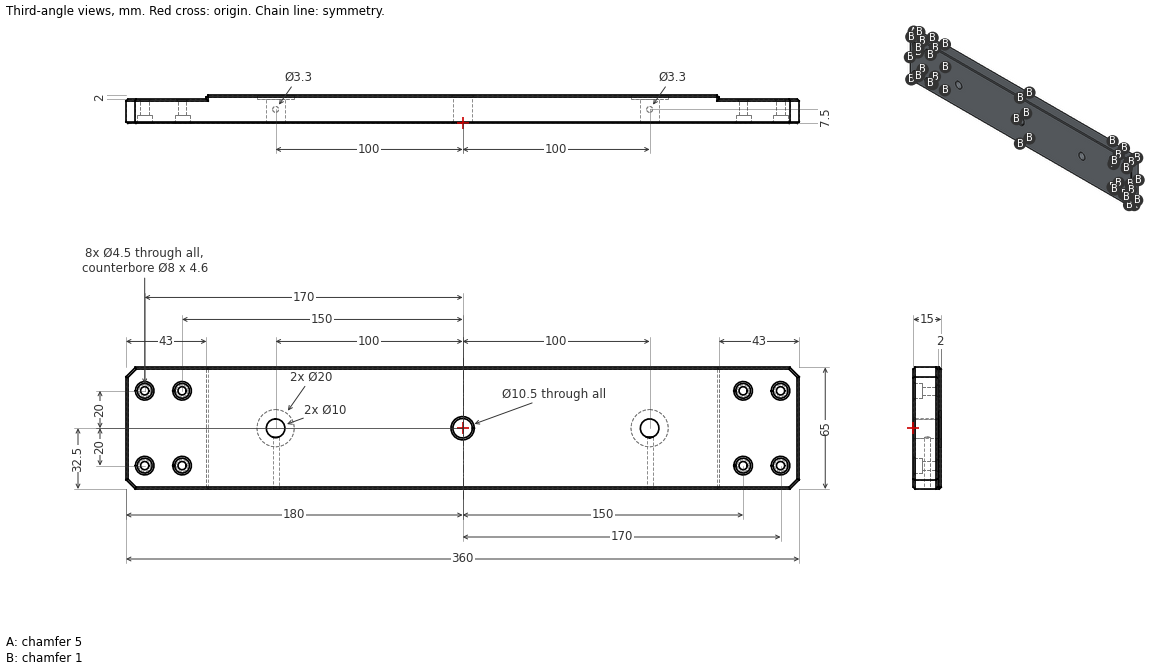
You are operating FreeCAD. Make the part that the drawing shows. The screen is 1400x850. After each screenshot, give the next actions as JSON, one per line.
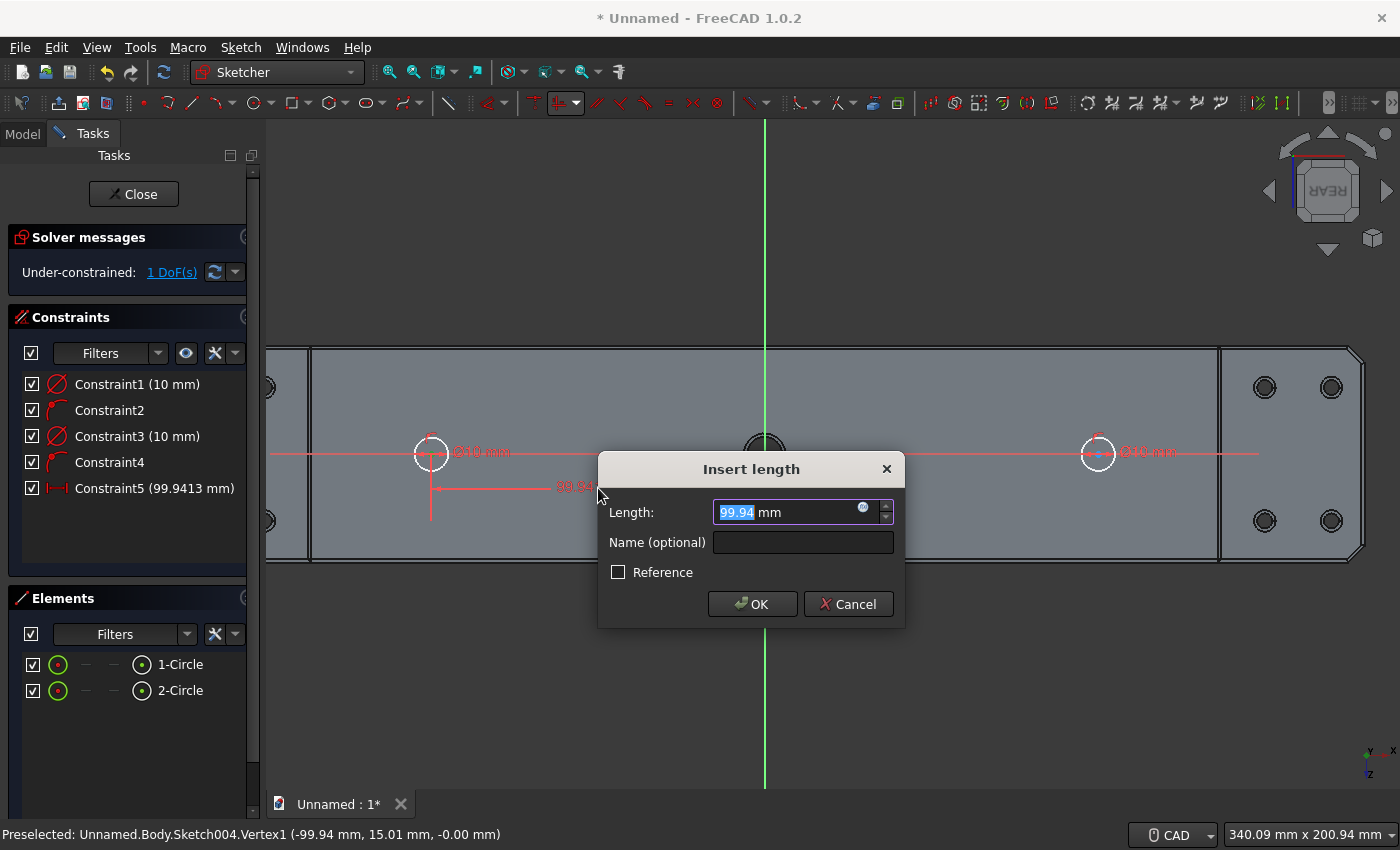
{"action": "type", "text": "100"}
{"action": "key", "text": "Return"}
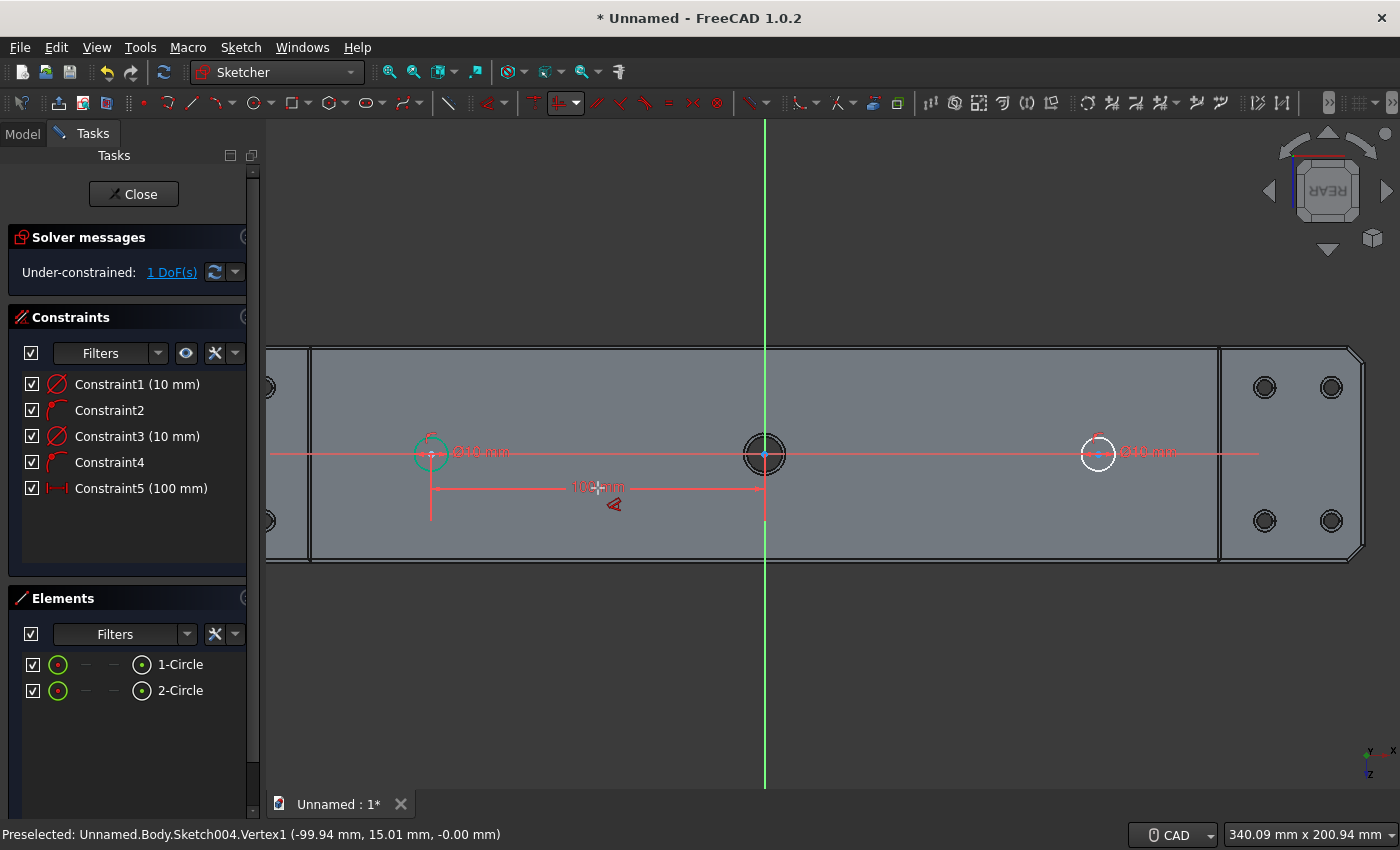
{"action": "left_click", "coordinate": [1098, 454]}
{"action": "left_click", "coordinate": [931, 488]}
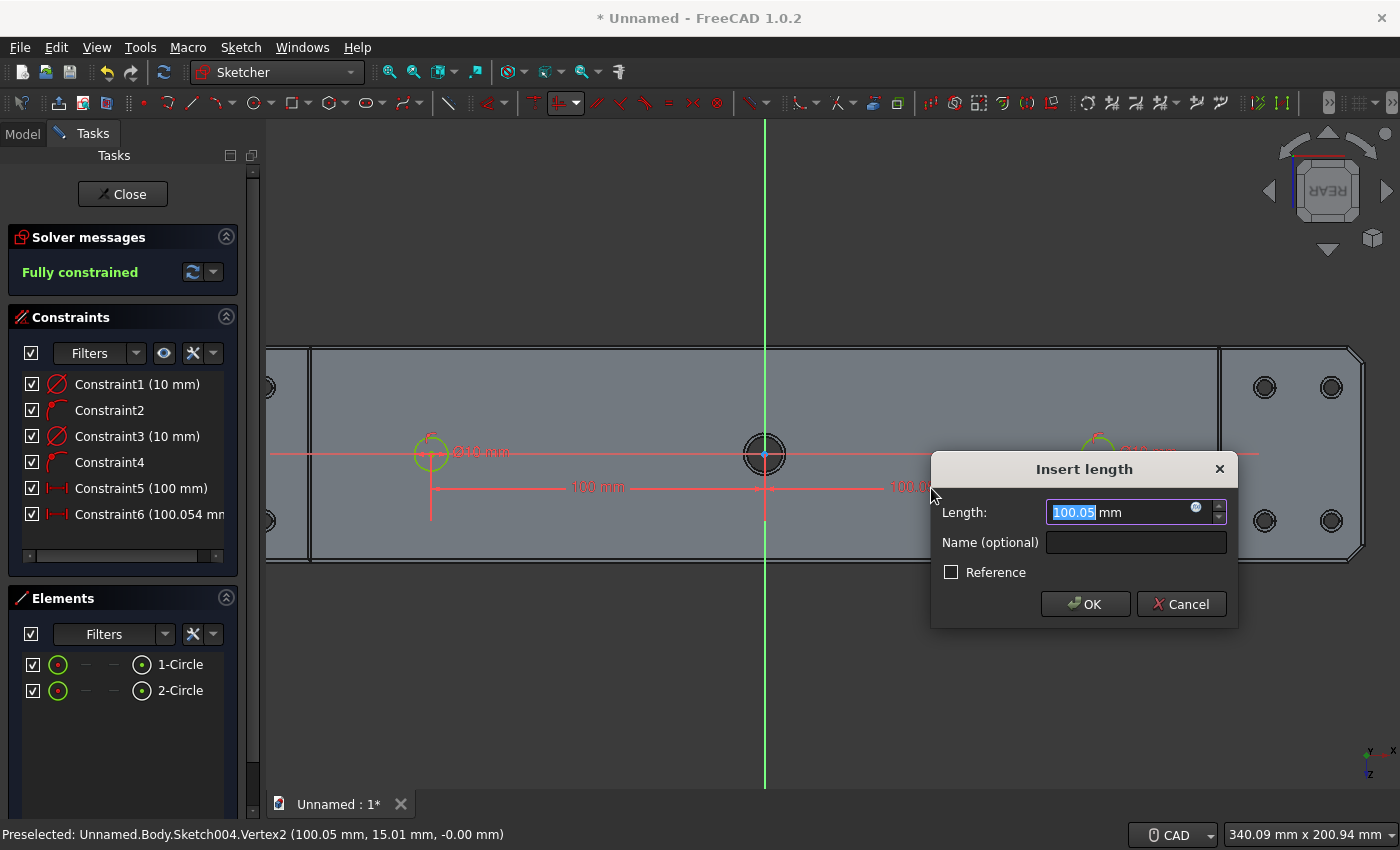
{"action": "type", "text": "100"}
{"action": "key", "text": "Return"}
{"action": "key", "text": "Escape"}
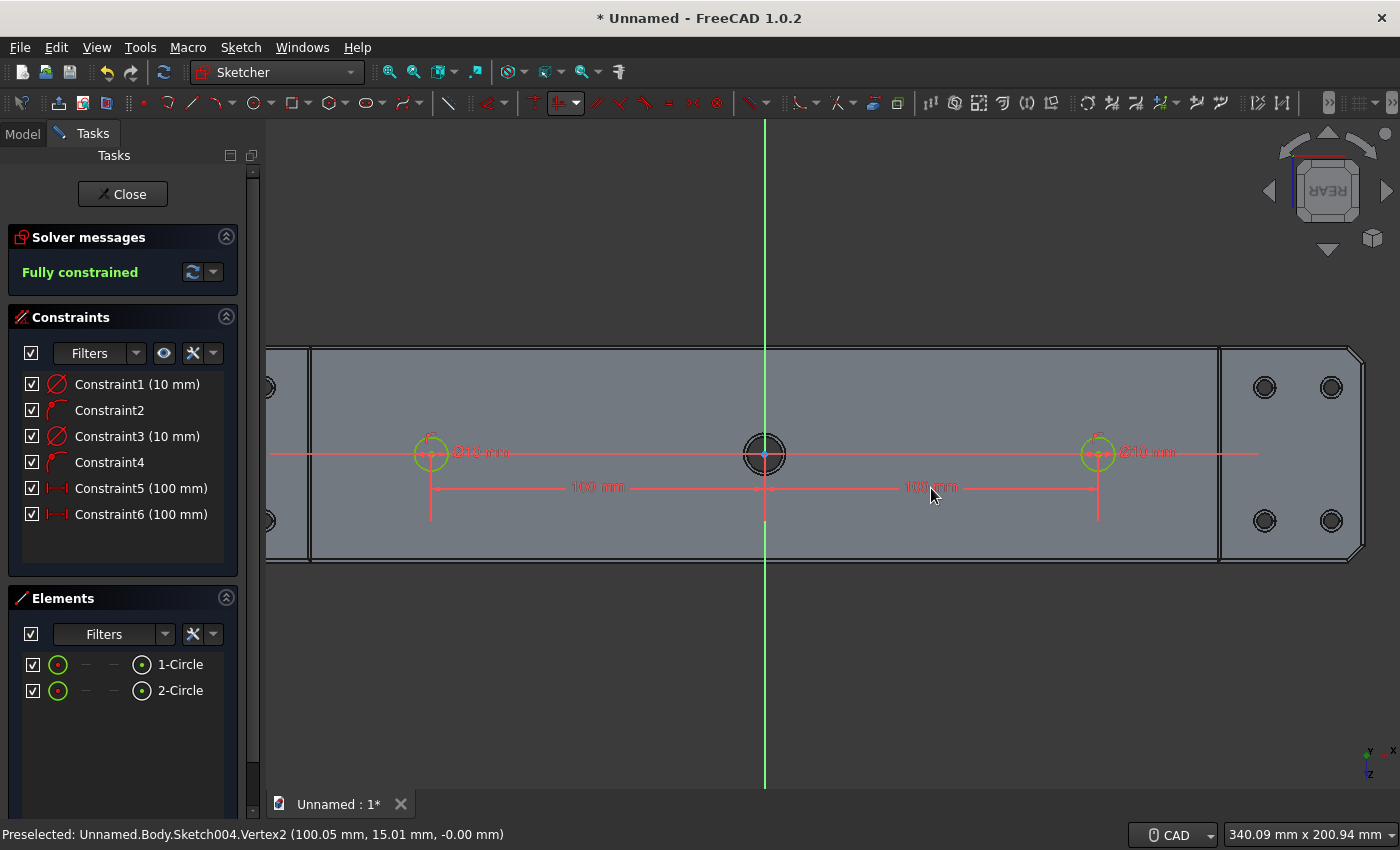
{"action": "left_click", "coordinate": [123, 194]}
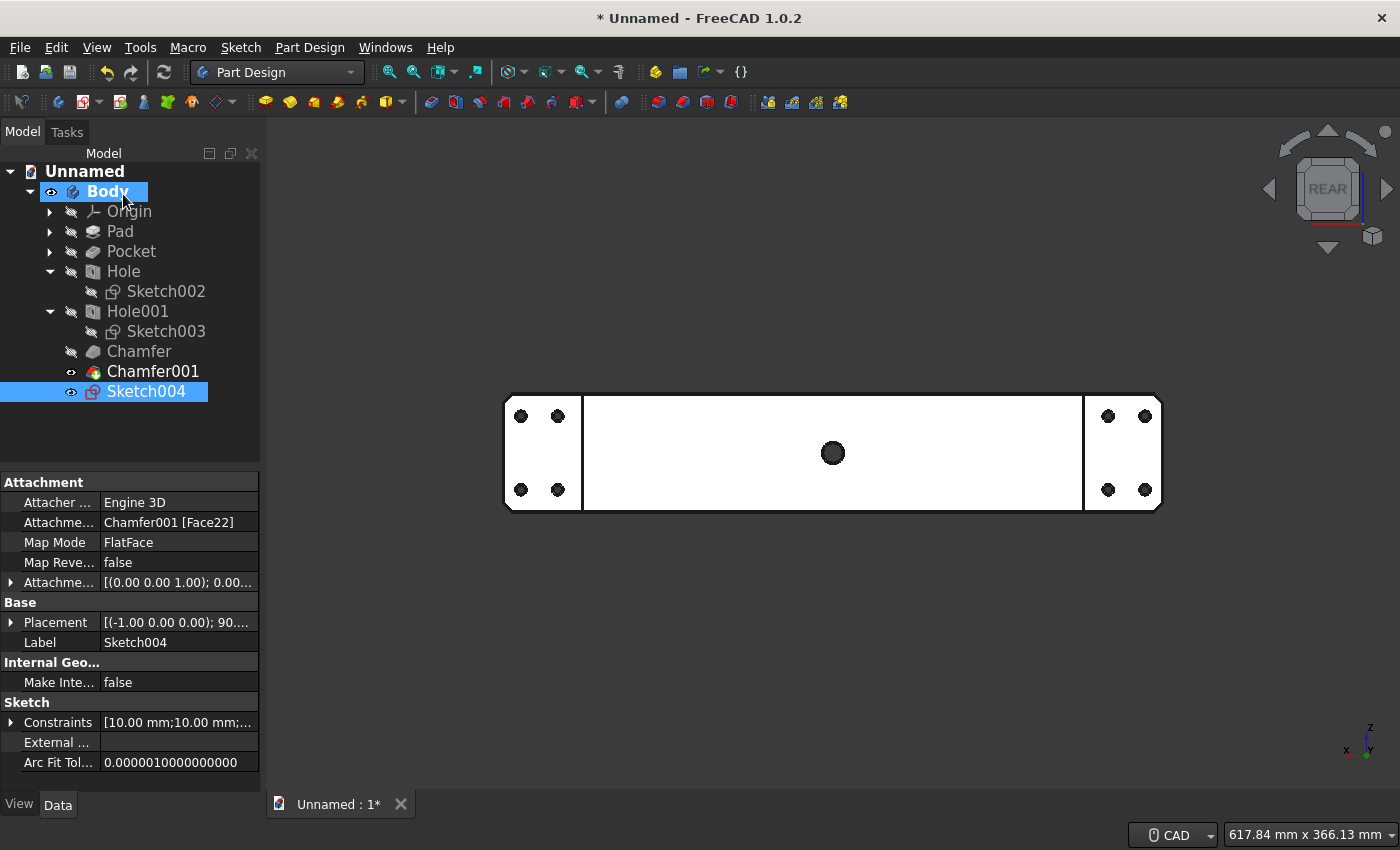
{"action": "left_click", "coordinate": [432, 102]}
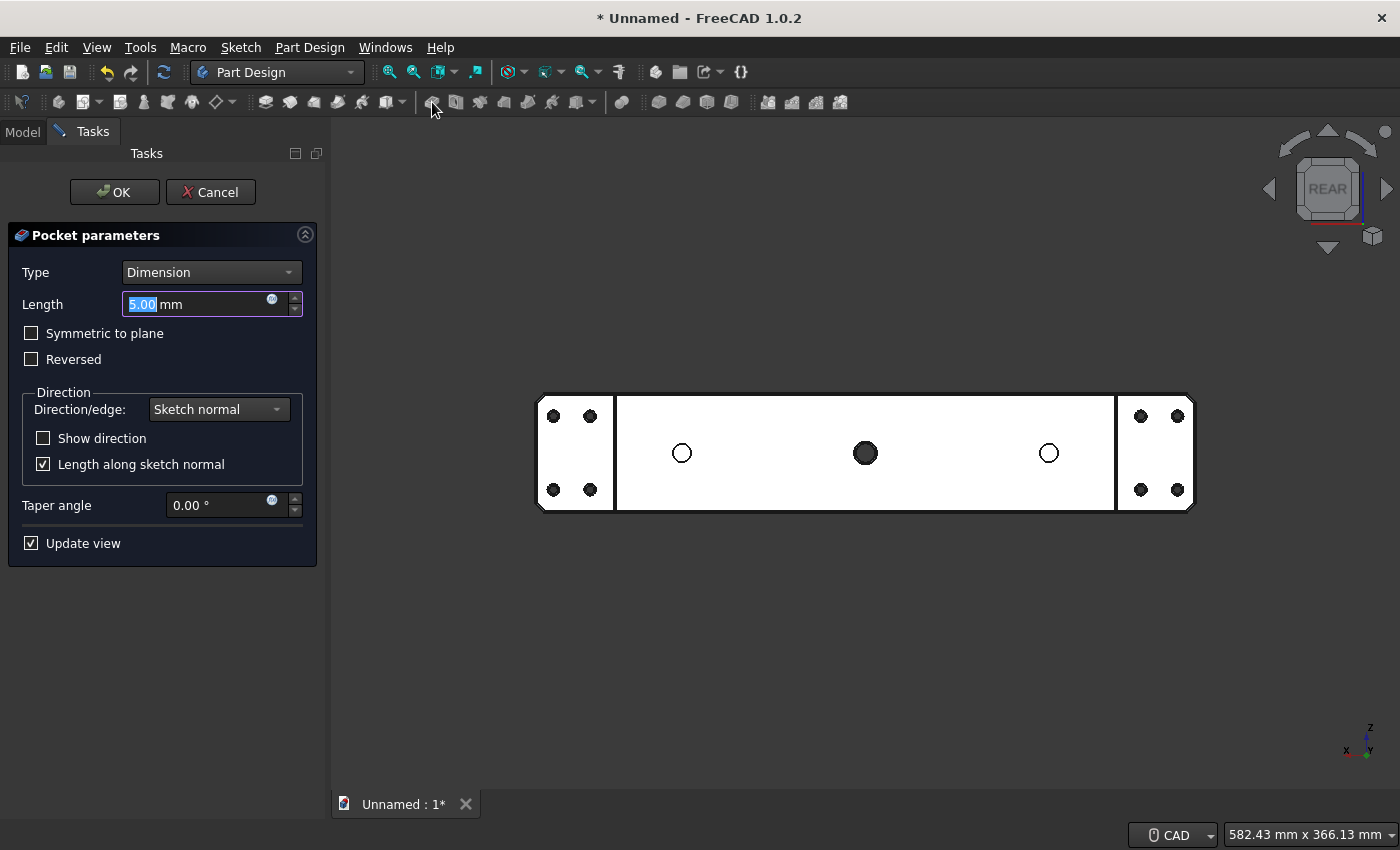
{"action": "left_click", "coordinate": [212, 272]}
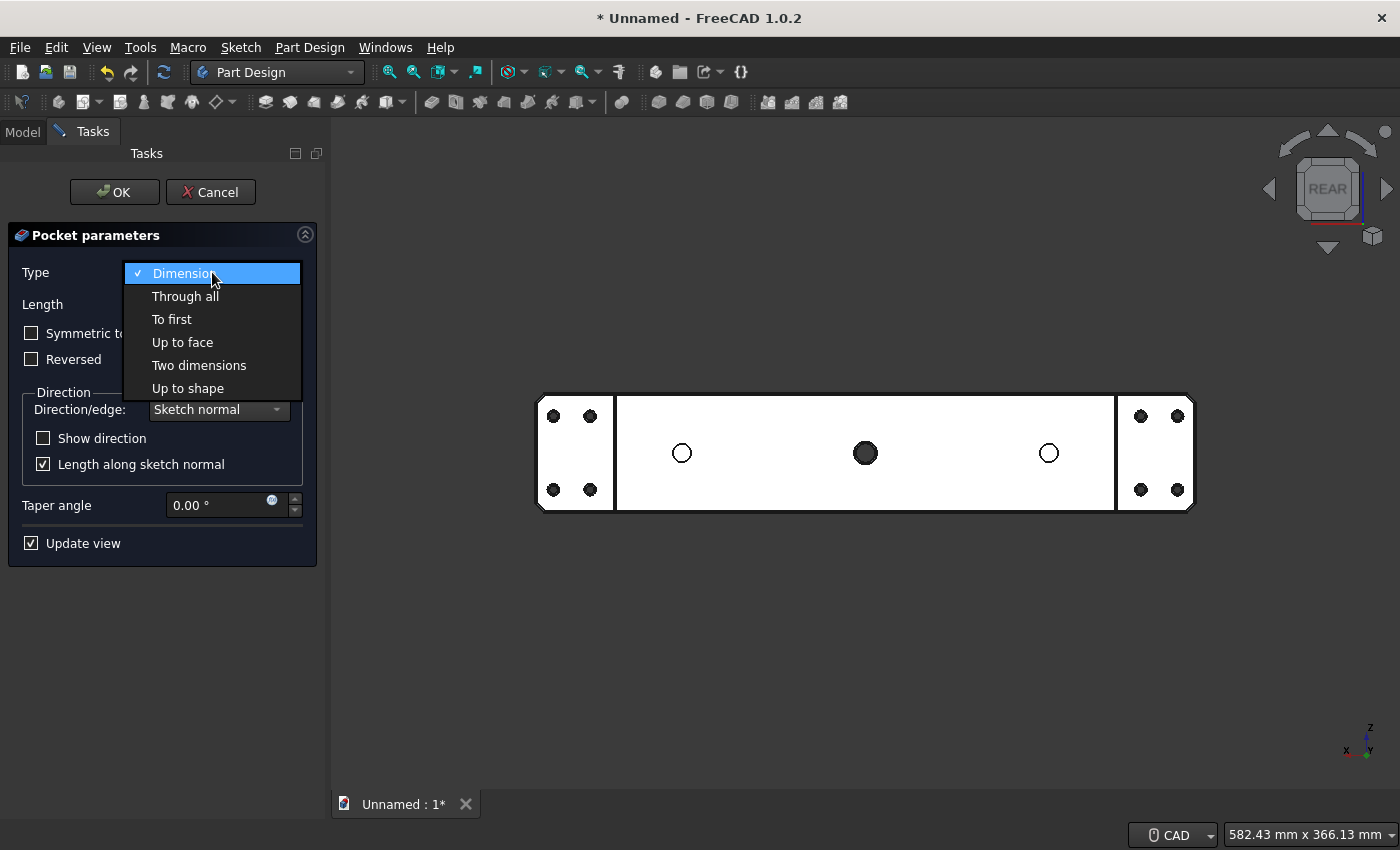
{"action": "left_click", "coordinate": [212, 296]}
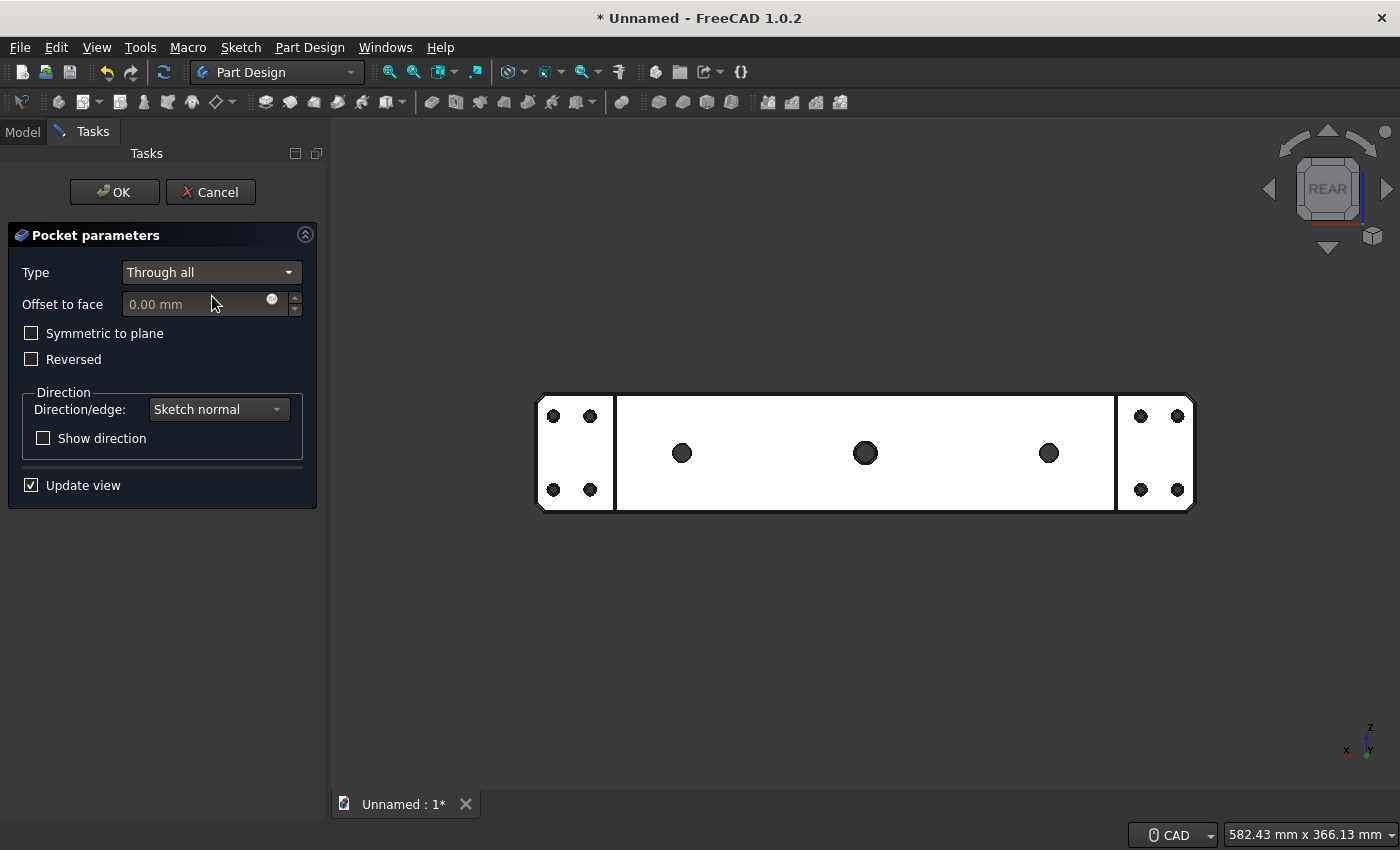
{"action": "left_click", "coordinate": [115, 192]}